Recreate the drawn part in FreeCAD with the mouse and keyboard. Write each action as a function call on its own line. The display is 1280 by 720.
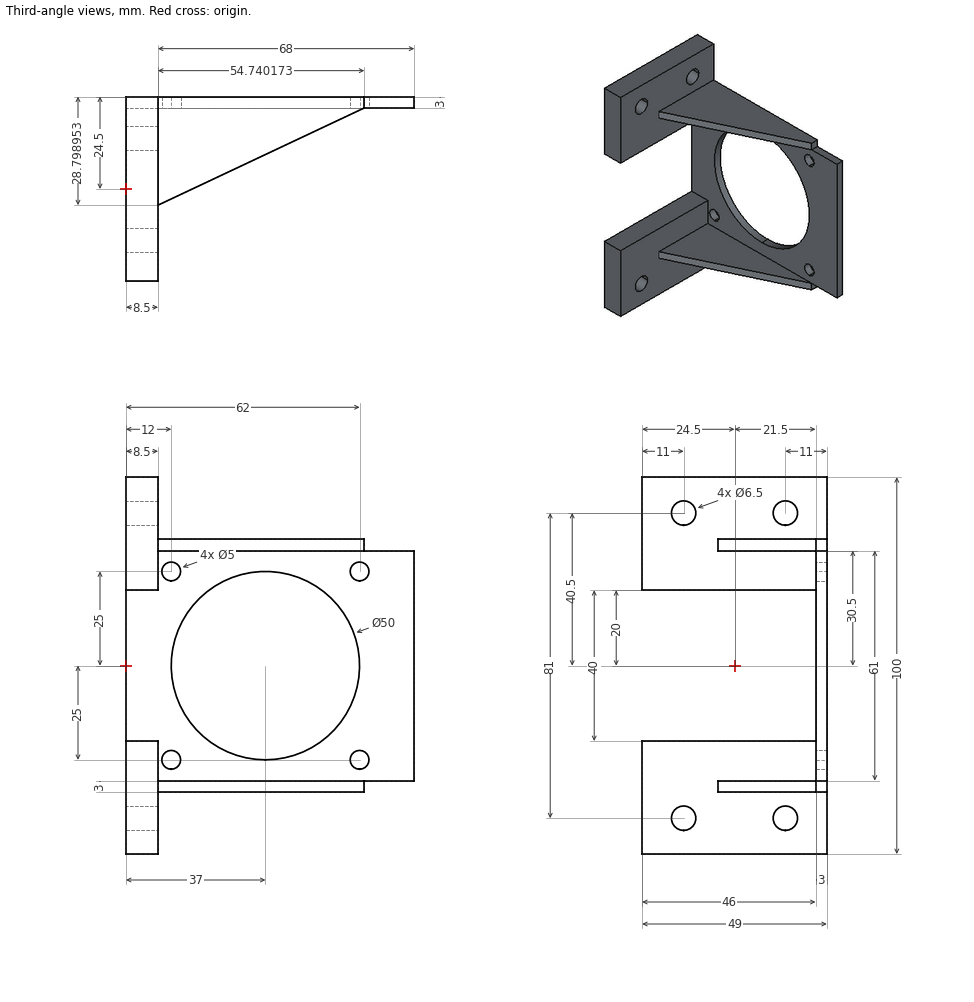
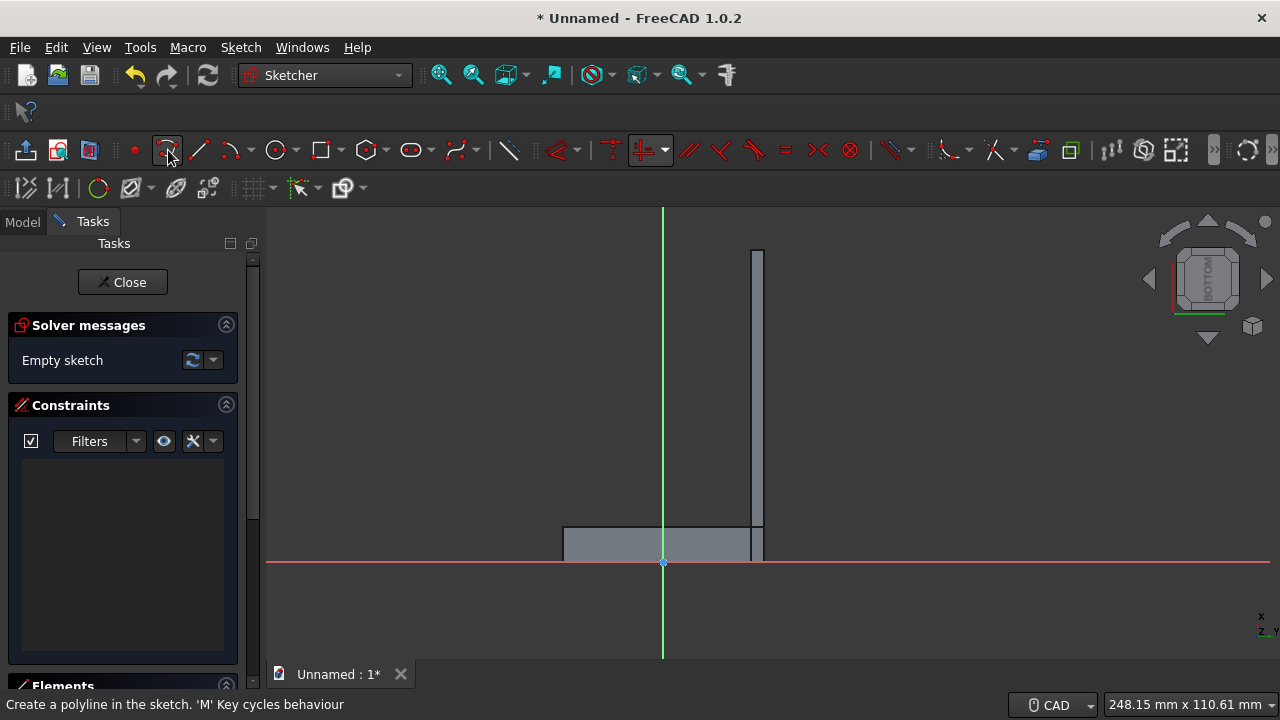
click(646, 527)
click(764, 527)
click(764, 304)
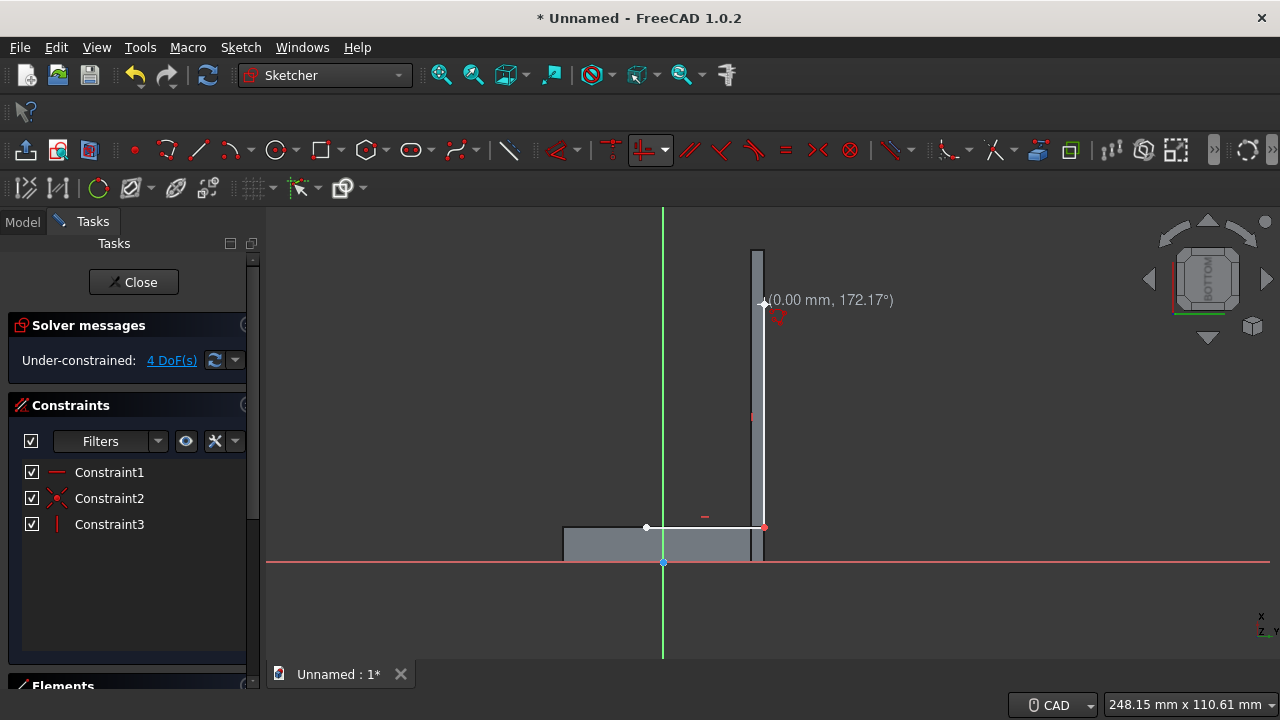
scroll(751, 304, up, 2)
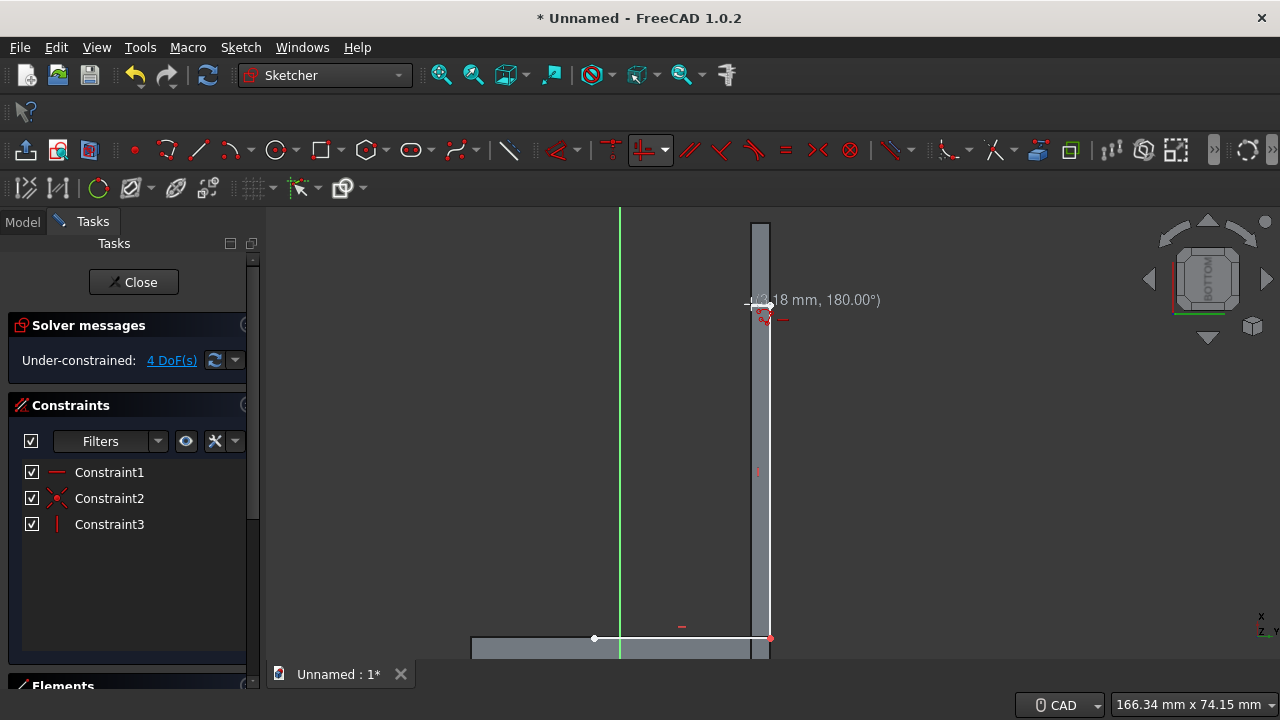
click(751, 304)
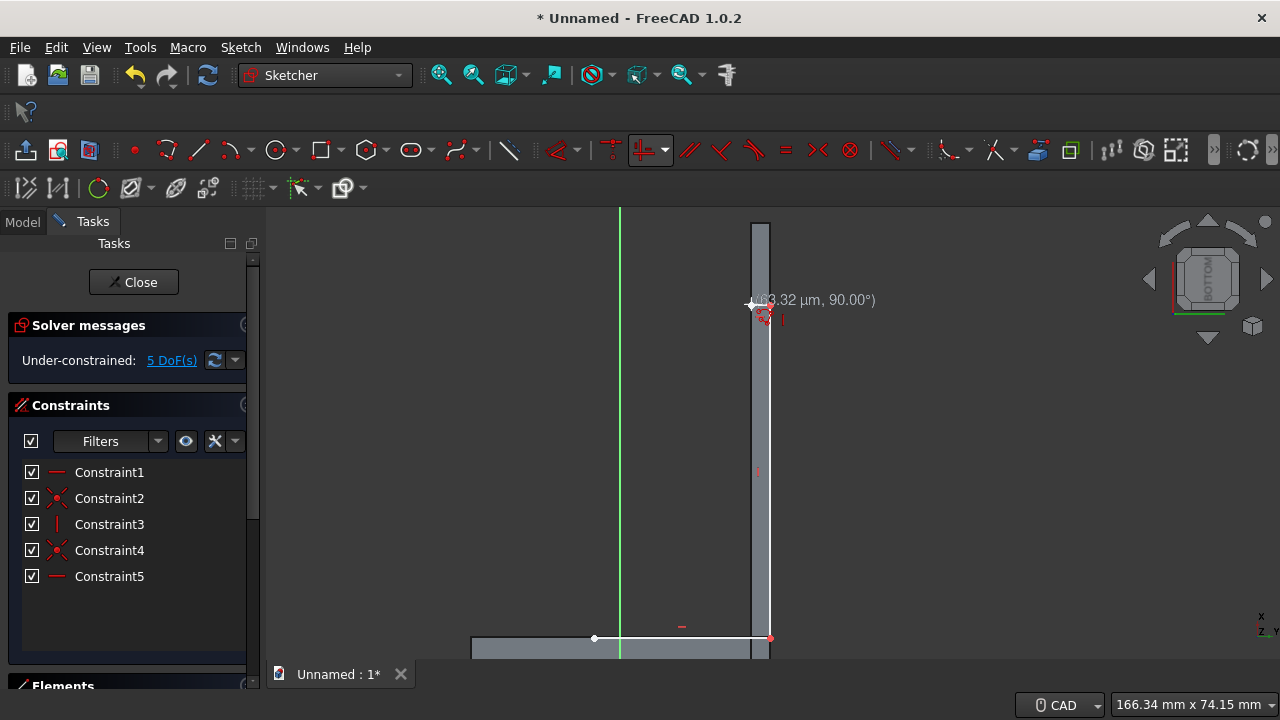
scroll(751, 304, down, 2)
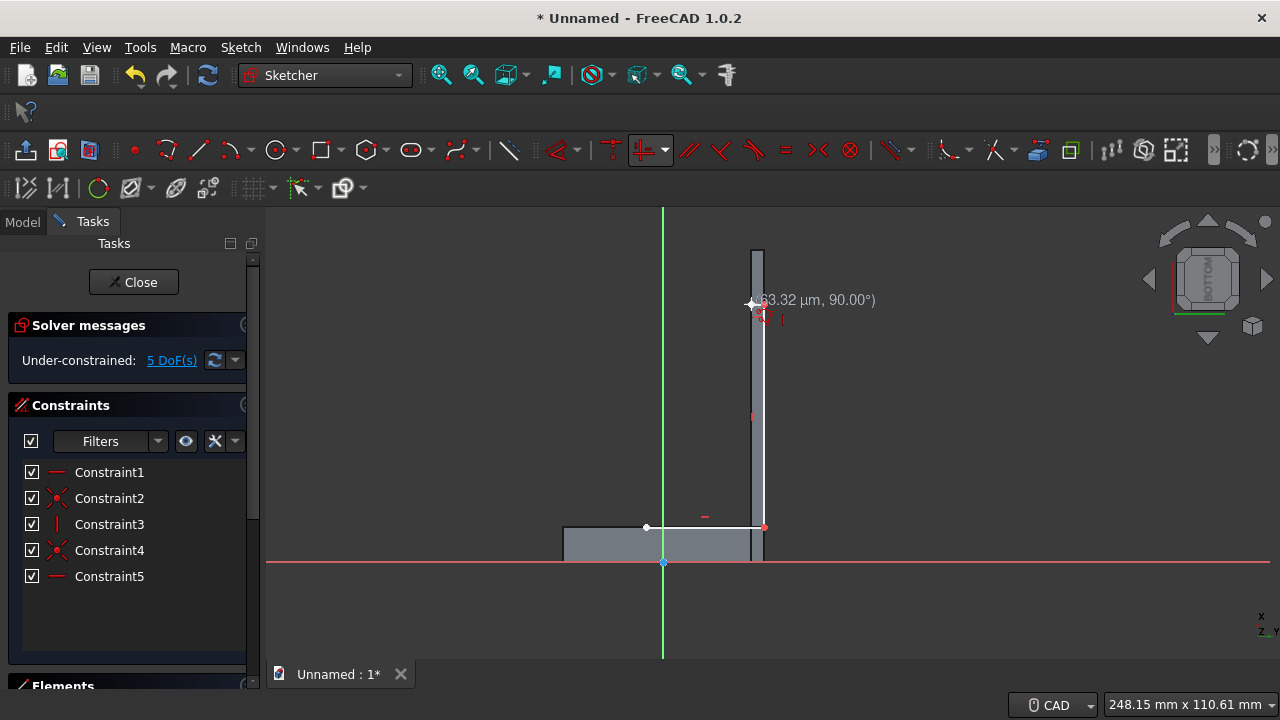
click(646, 528)
key(Escape)
key(Escape)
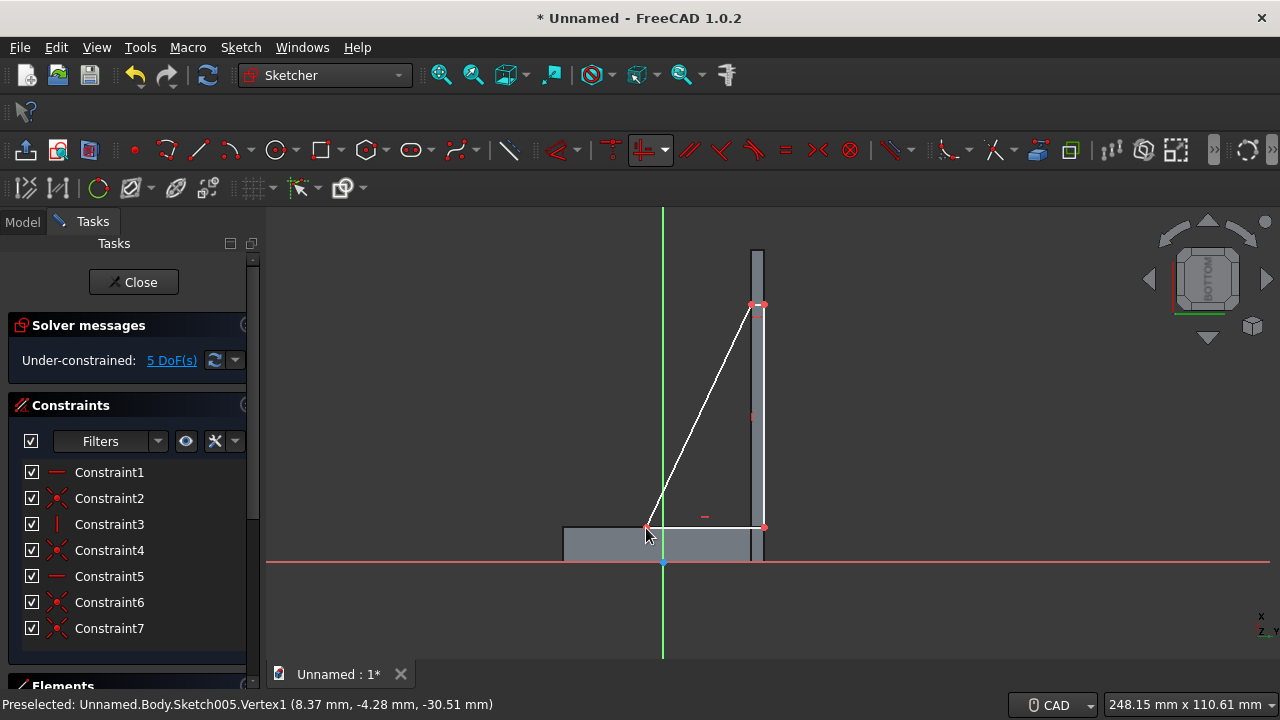
click(556, 150)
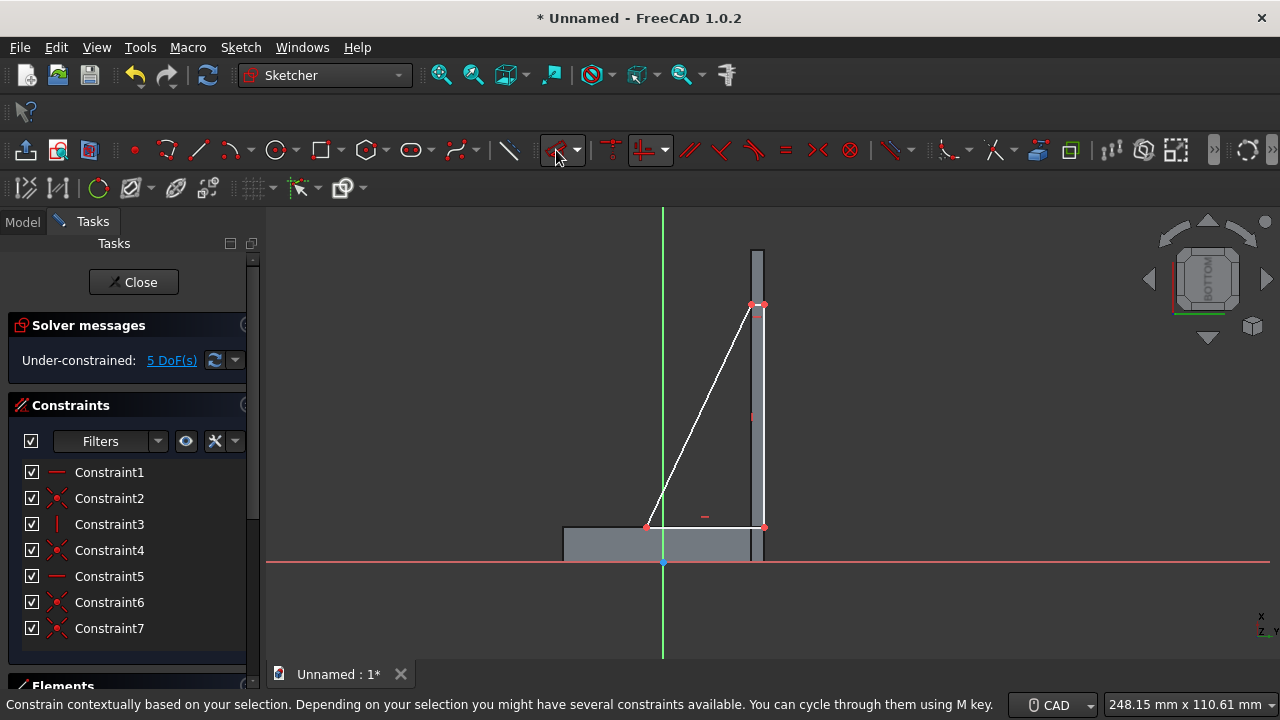
scroll(758, 305, up, 6)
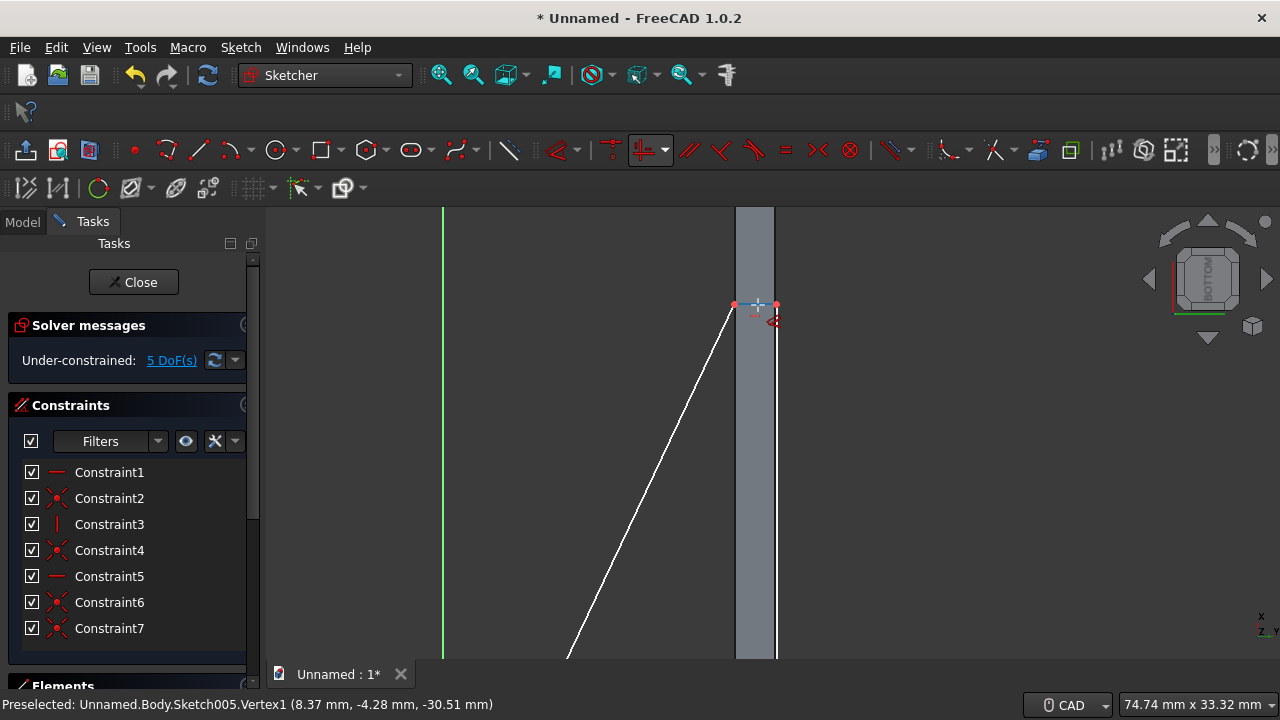
click(755, 304)
click(755, 270)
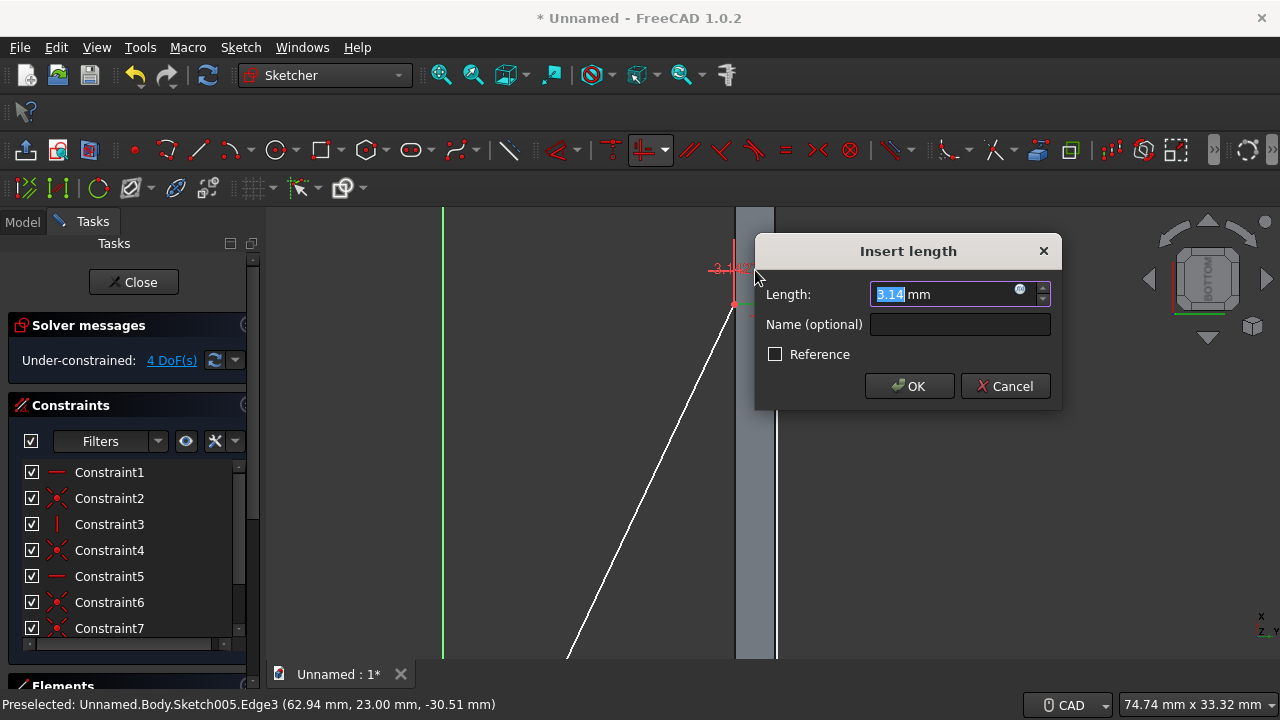
text(3)
key(Return)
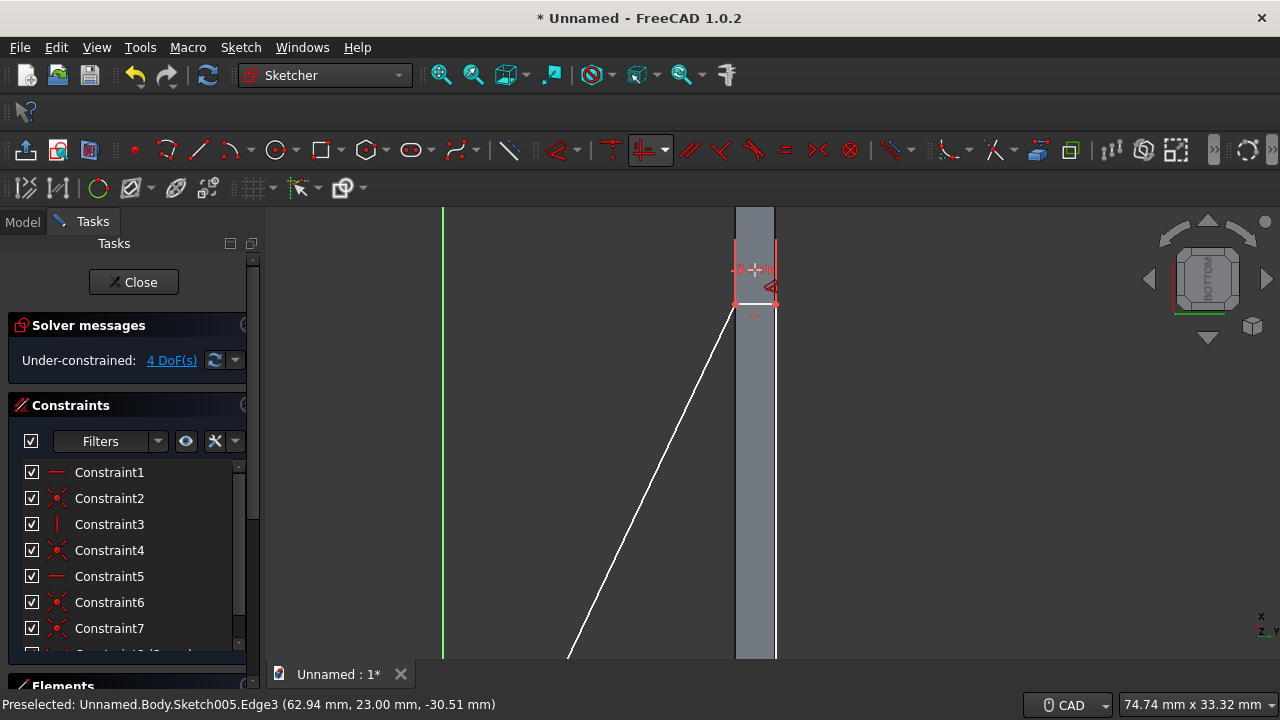
scroll(758, 305, down, 6)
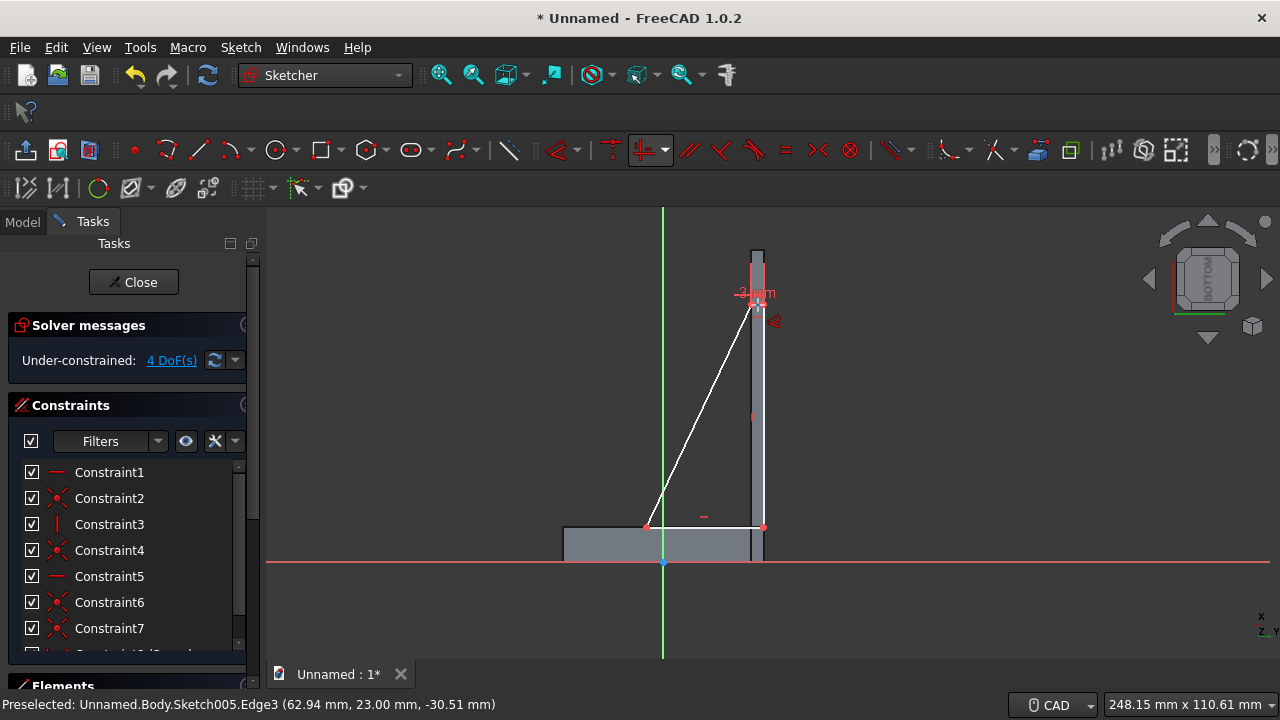
click(646, 528)
click(612, 545)